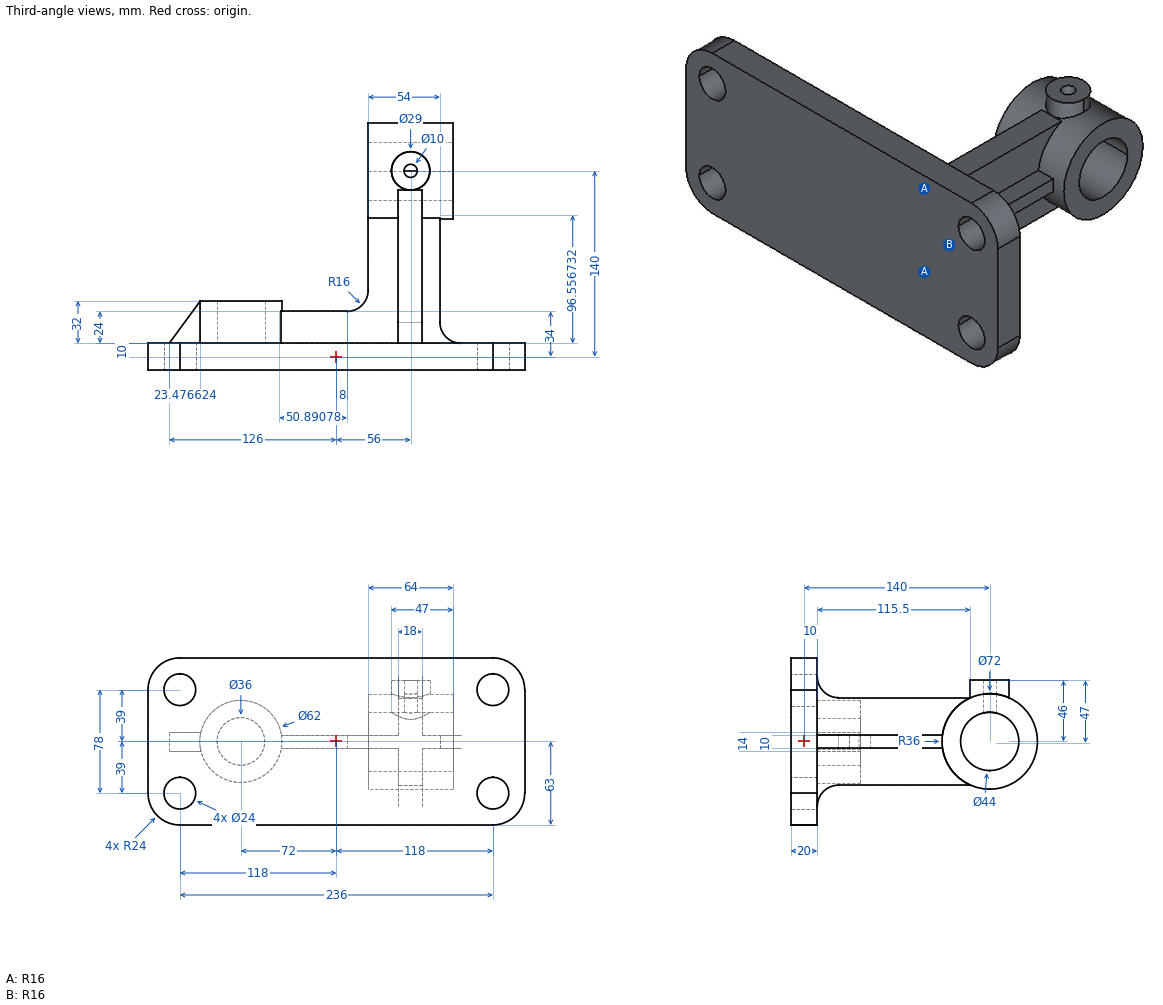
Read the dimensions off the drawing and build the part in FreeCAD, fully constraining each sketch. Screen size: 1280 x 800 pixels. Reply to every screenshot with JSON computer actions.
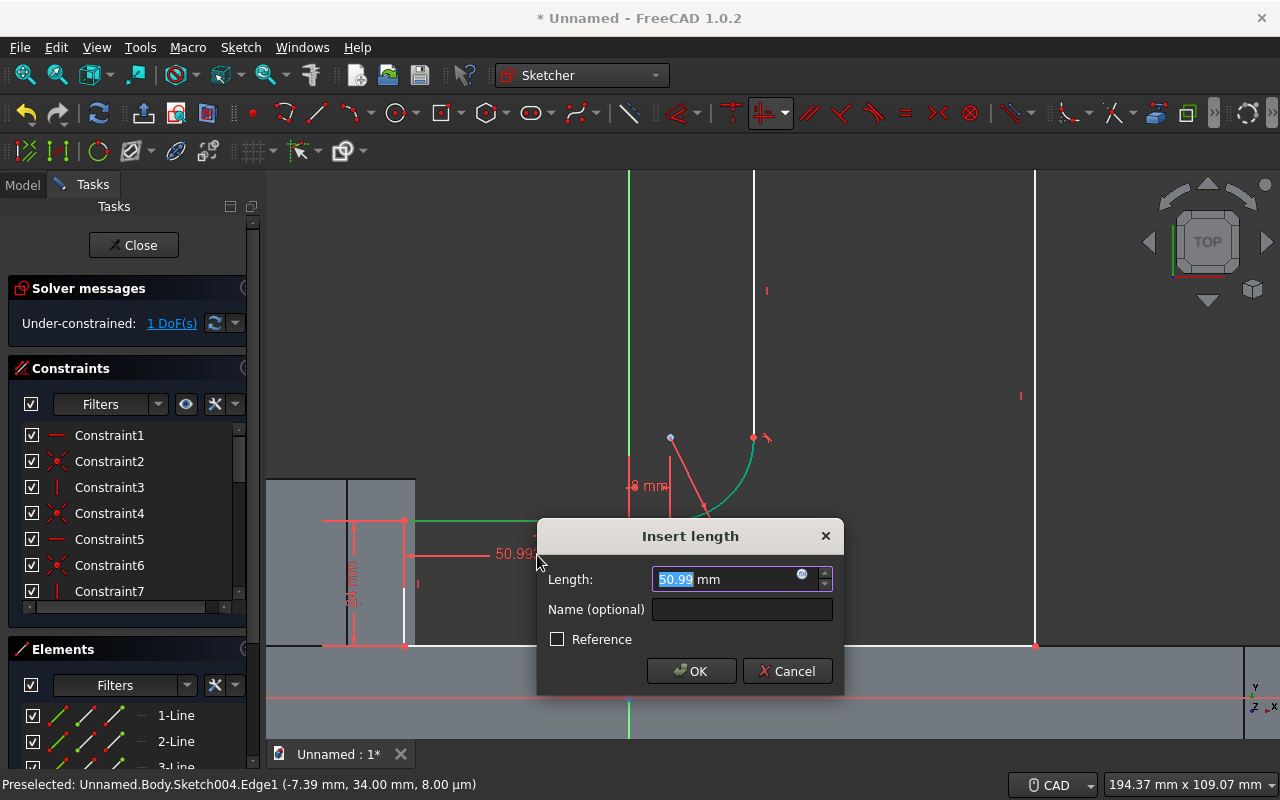
{"action": "type", "text": "50.89078"}
{"action": "key", "text": "Return"}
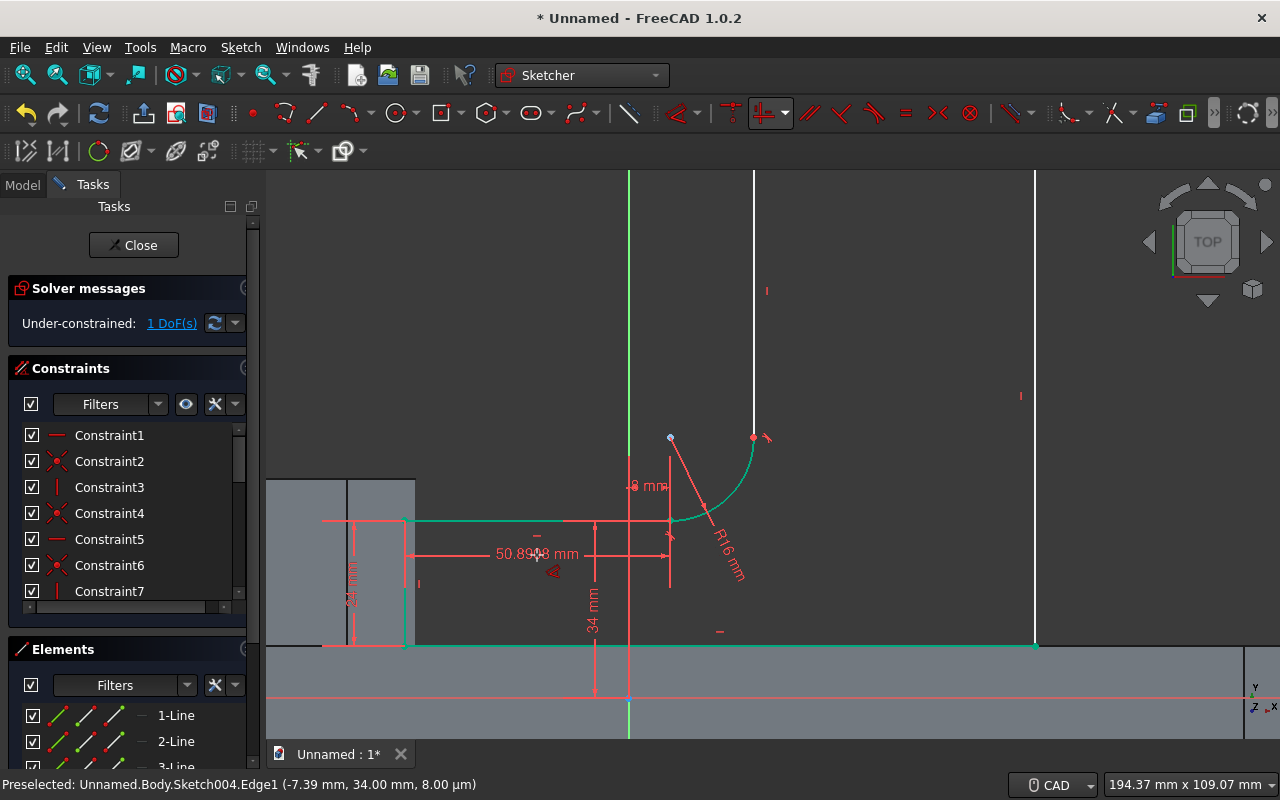
{"action": "left_click", "coordinate": [1035, 496]}
{"action": "left_click", "coordinate": [1069, 422]}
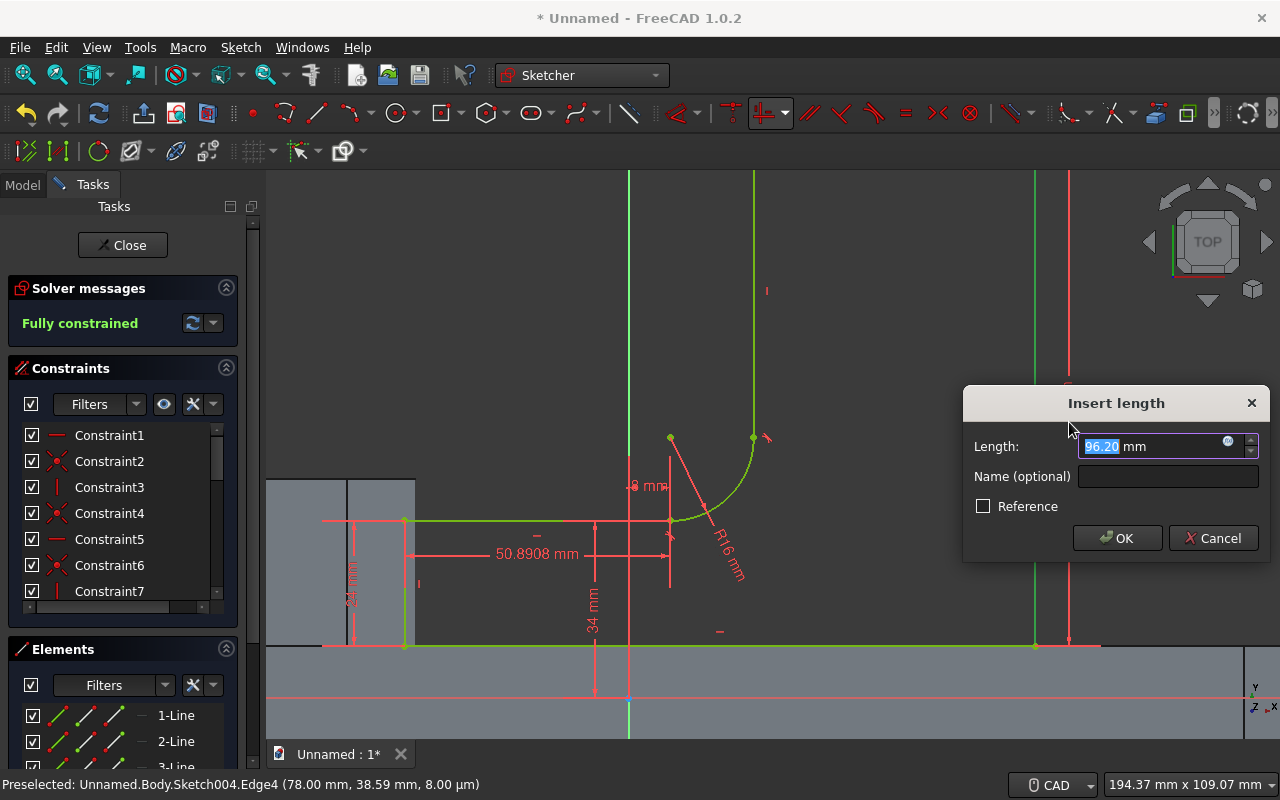
{"action": "type", "text": "96.556732"}
{"action": "key", "text": "Return"}
{"action": "key", "text": "Escape"}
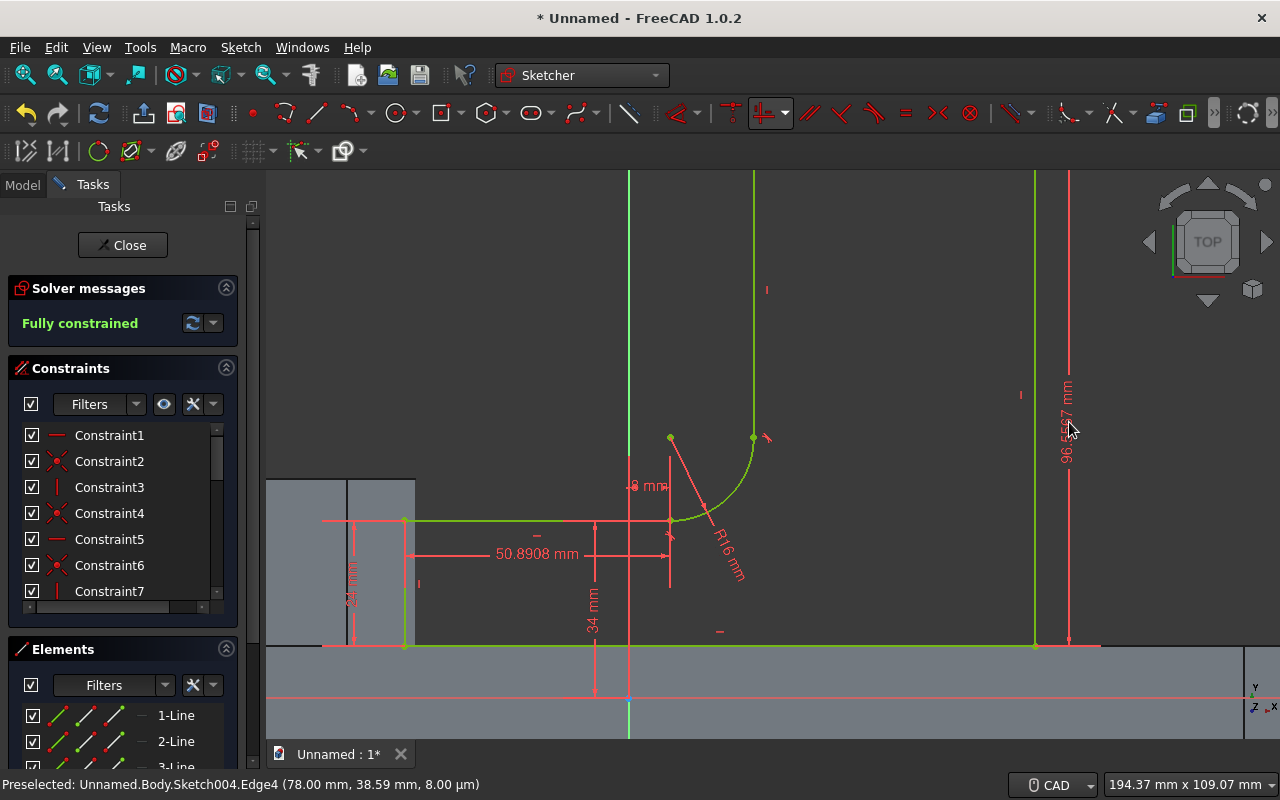
{"action": "left_click", "coordinate": [123, 245]}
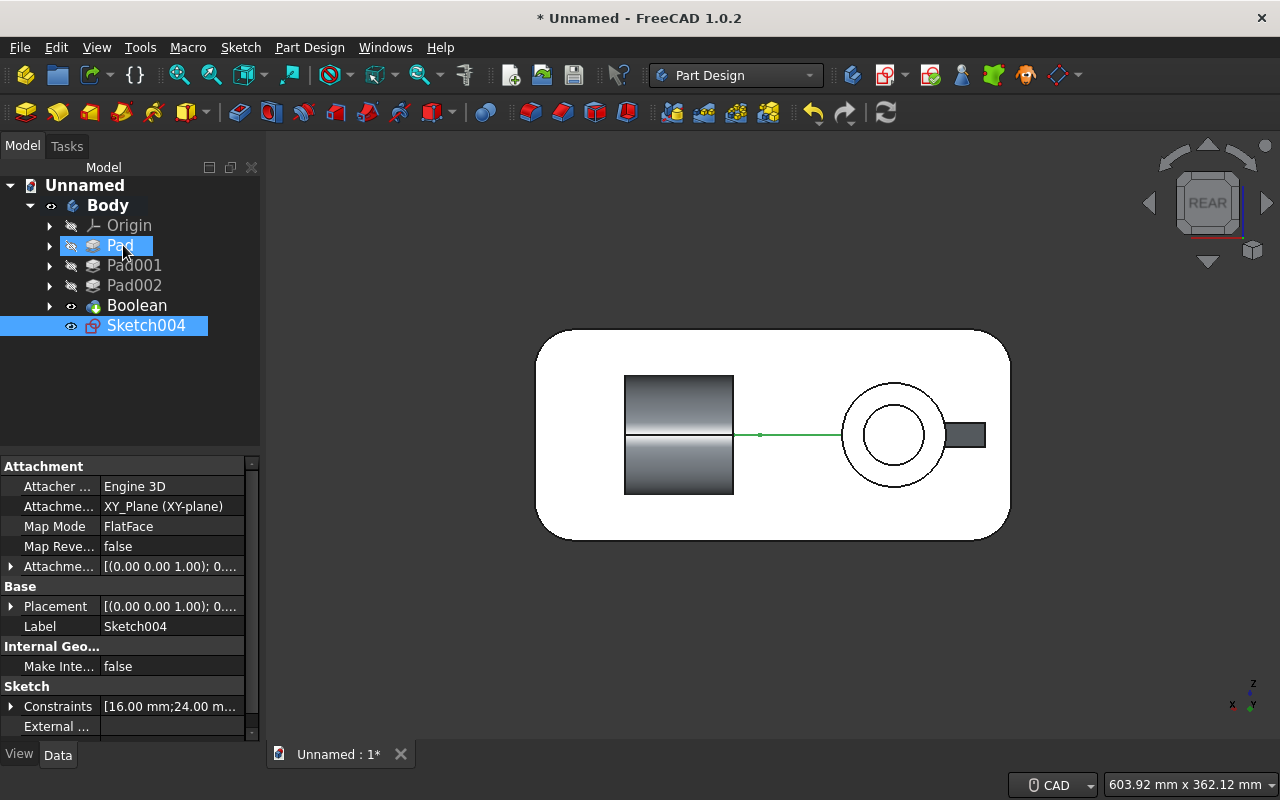
{"action": "left_click", "coordinate": [26, 112]}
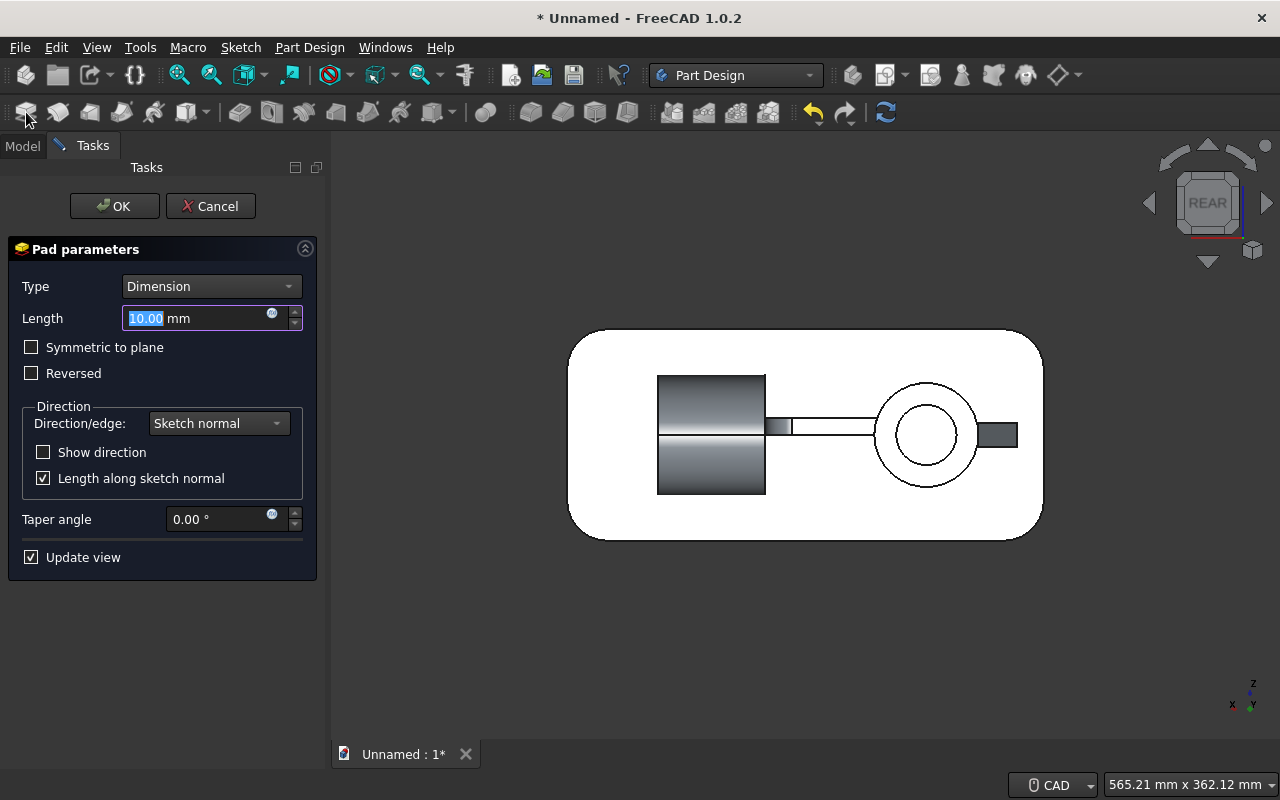
{"action": "type", "text": "10"}
{"action": "key", "text": "Tab"}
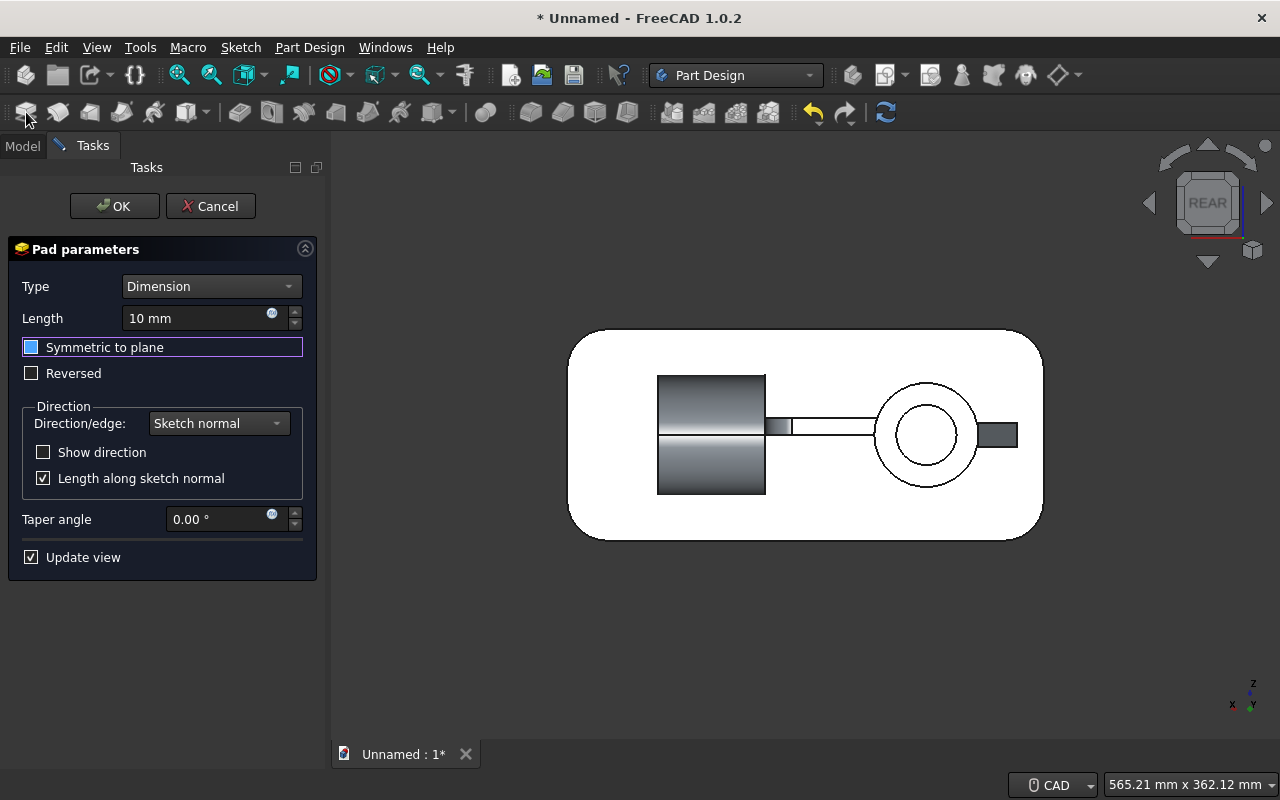
{"action": "left_click", "coordinate": [30, 347]}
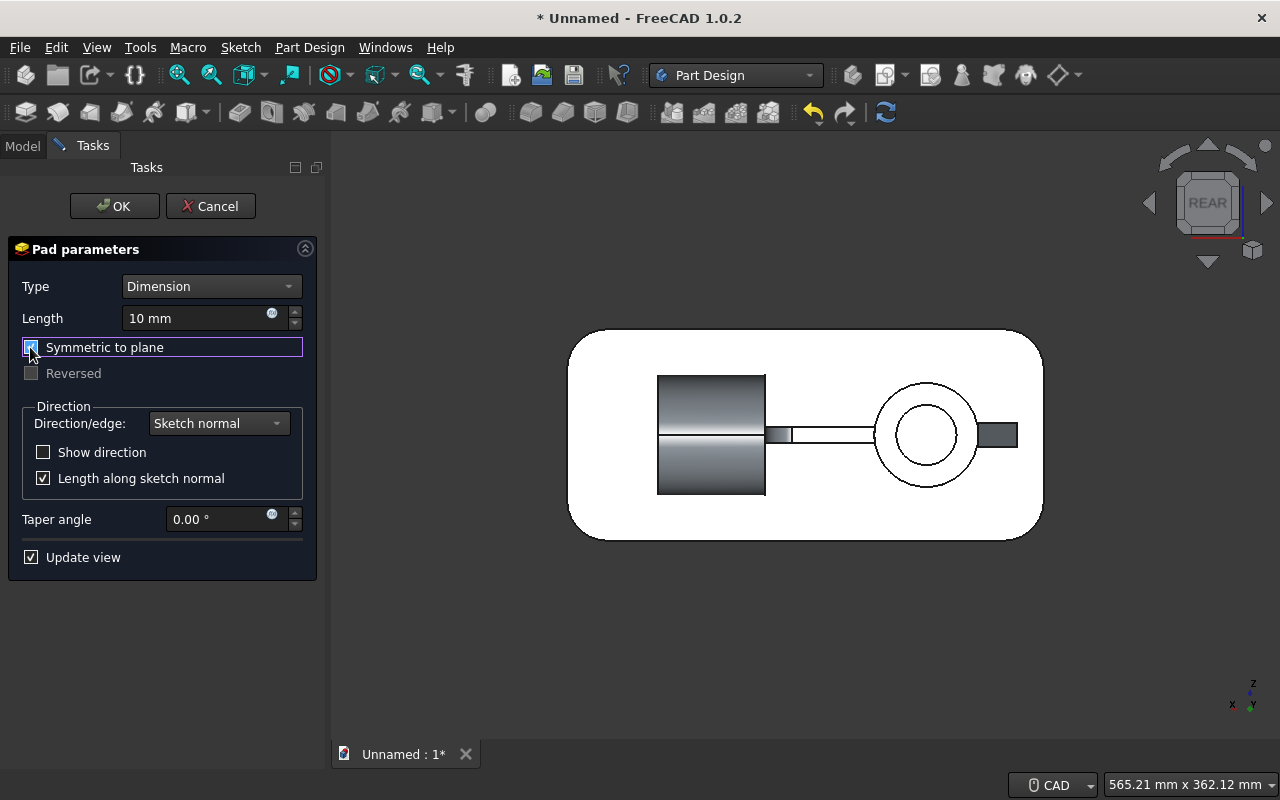
{"action": "left_click", "coordinate": [115, 206]}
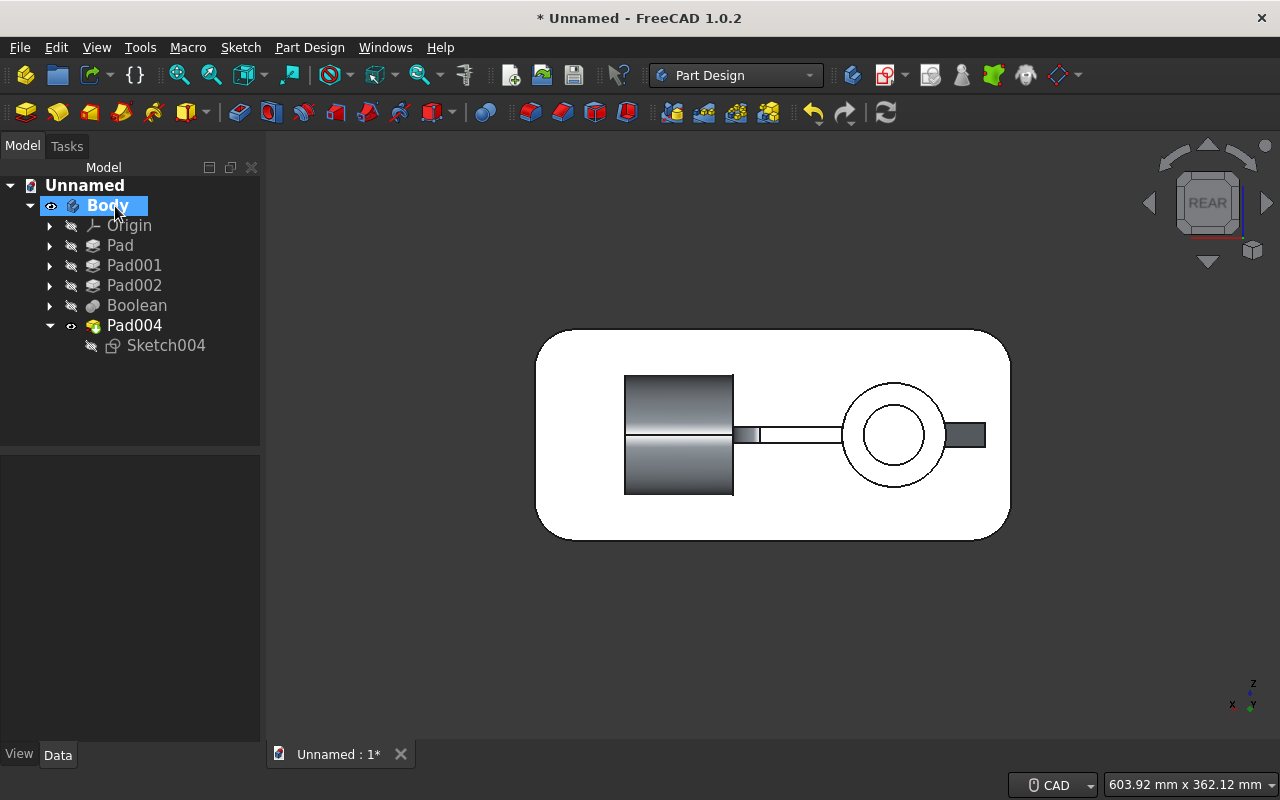
{"action": "left_click", "coordinate": [886, 76]}